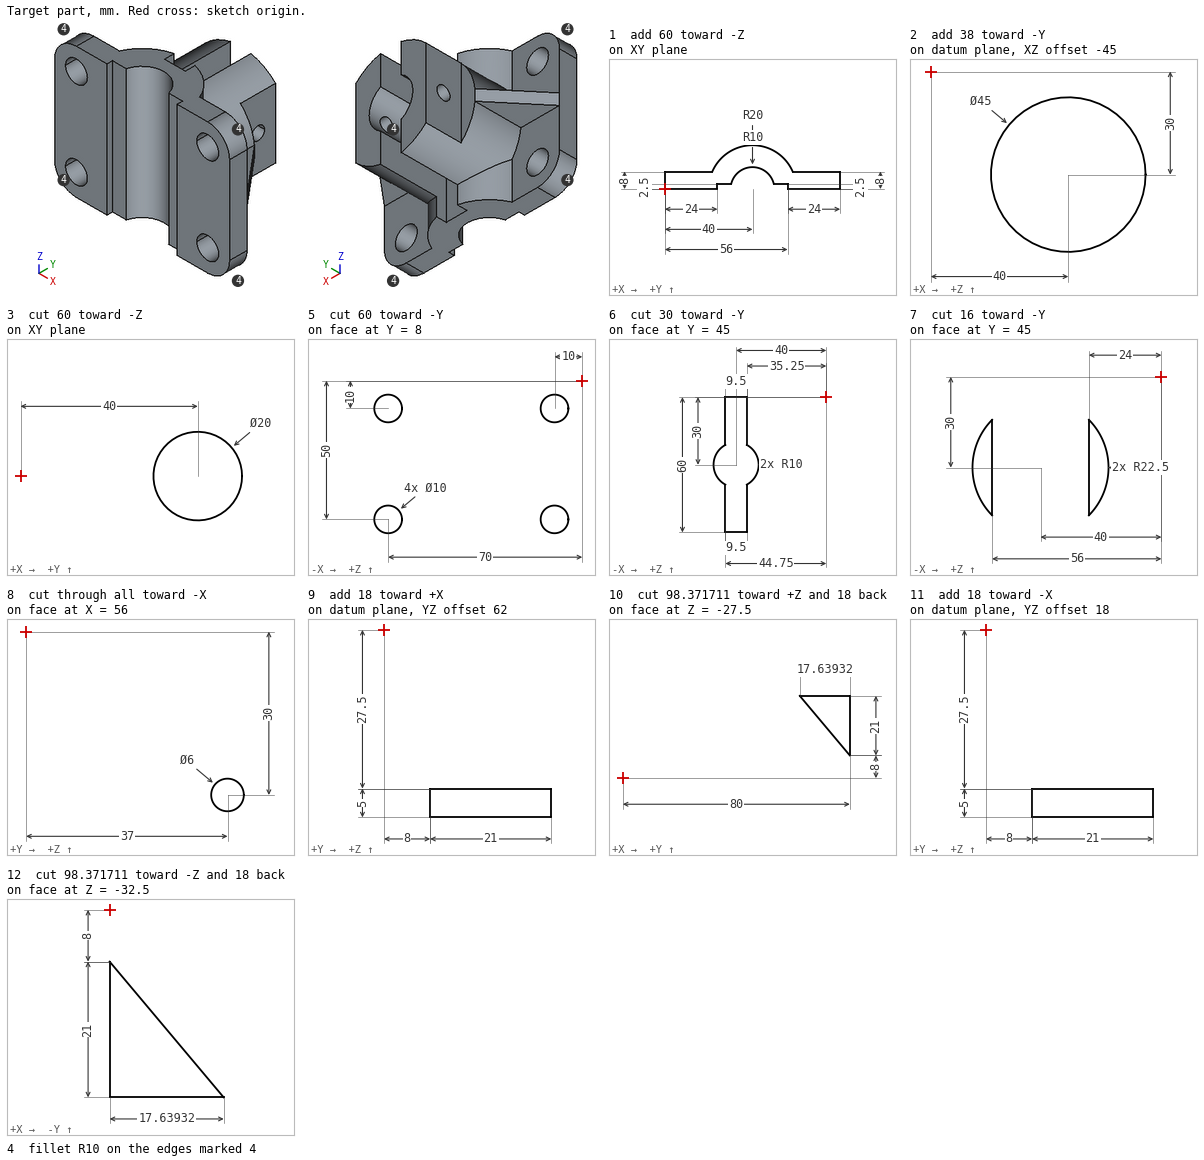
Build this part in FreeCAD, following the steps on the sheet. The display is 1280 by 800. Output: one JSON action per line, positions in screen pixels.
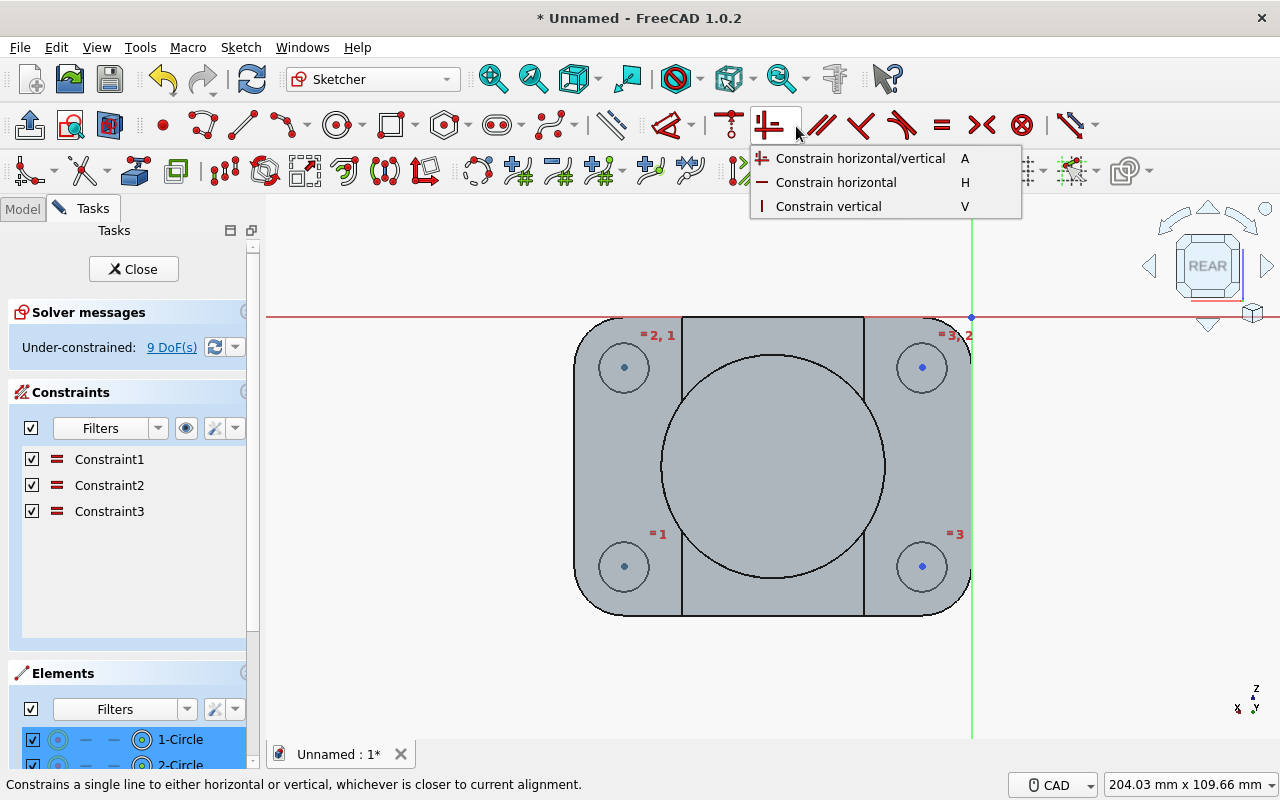
{"action": "left_click", "coordinate": [886, 206]}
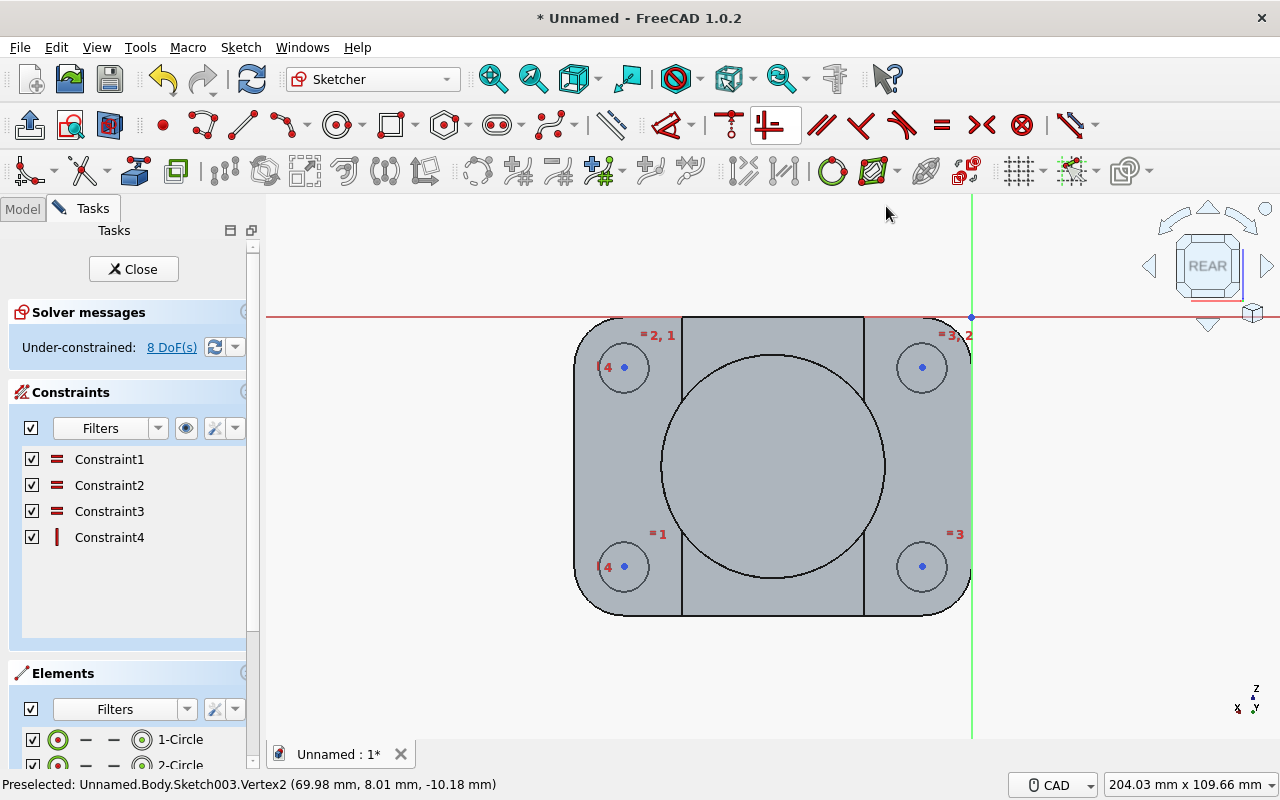
{"action": "left_click", "coordinate": [624, 368]}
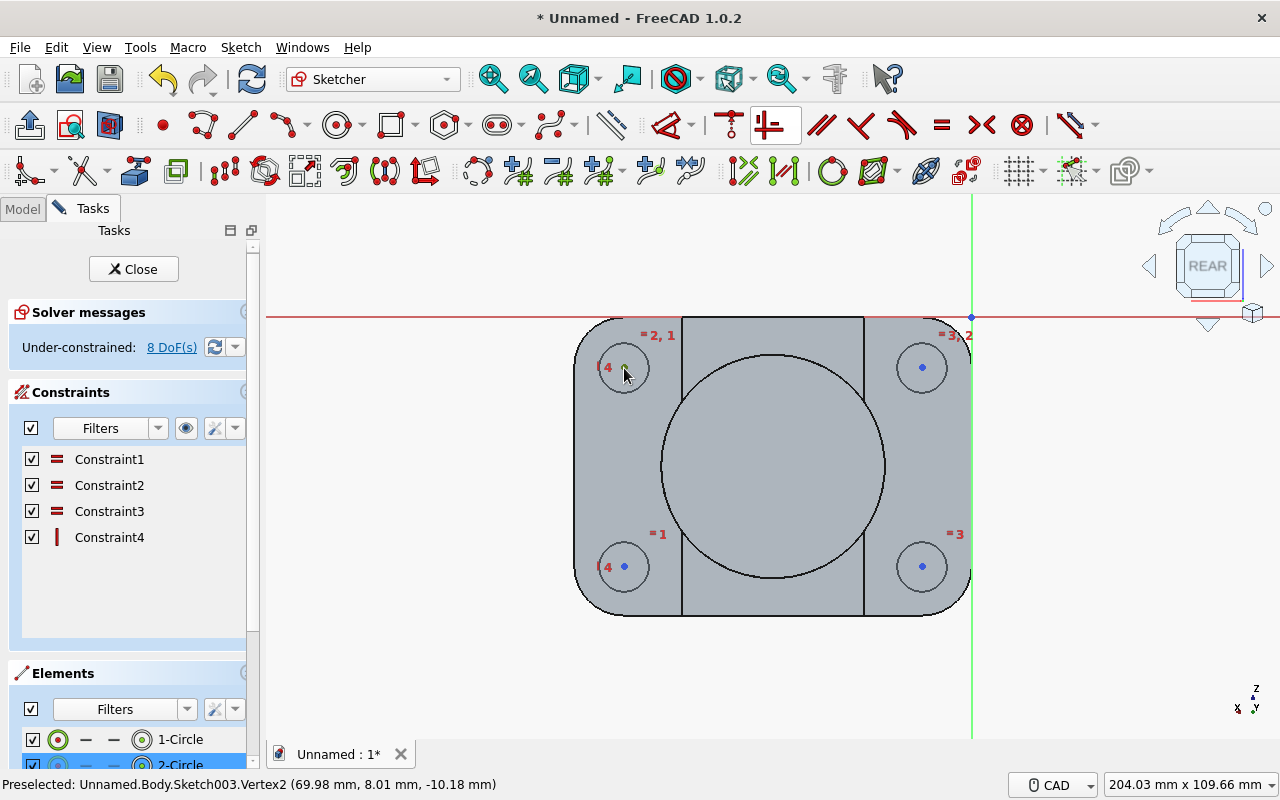
{"action": "left_click", "coordinate": [922, 368]}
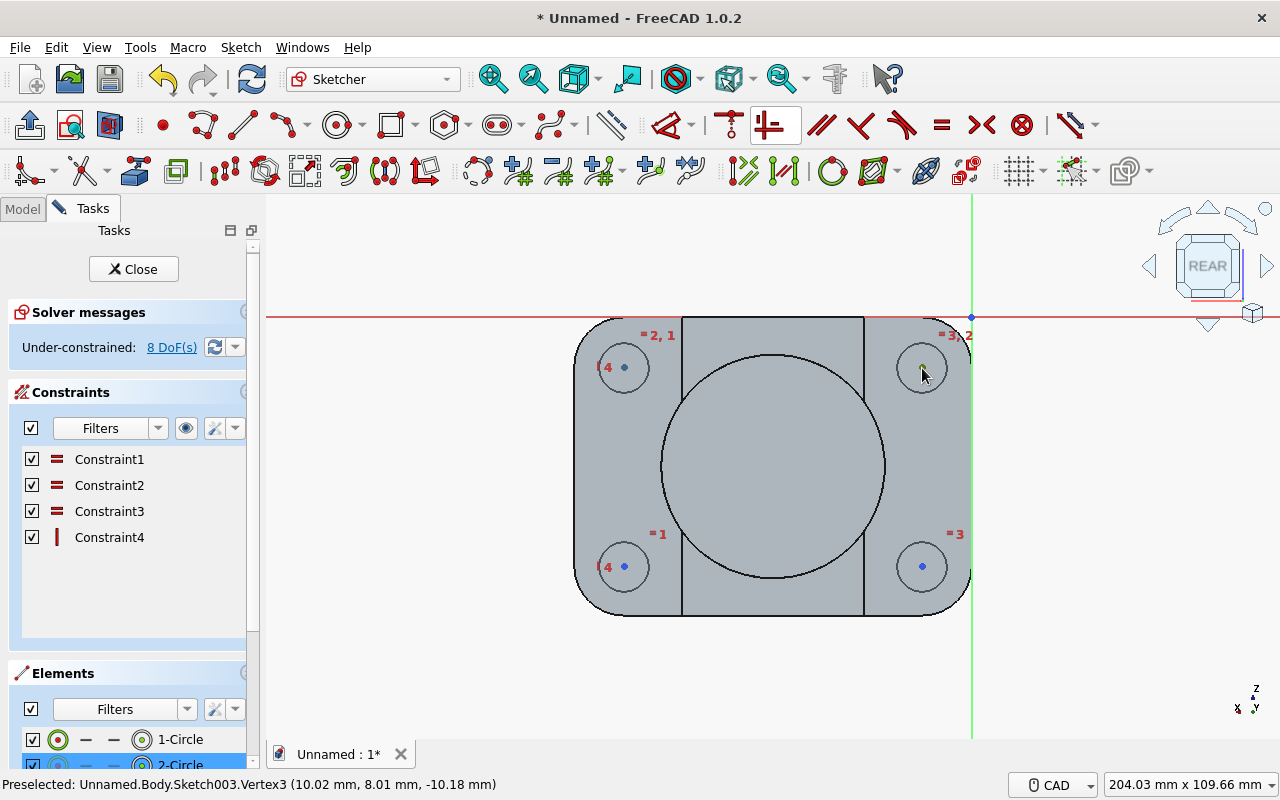
{"action": "left_click", "coordinate": [796, 126]}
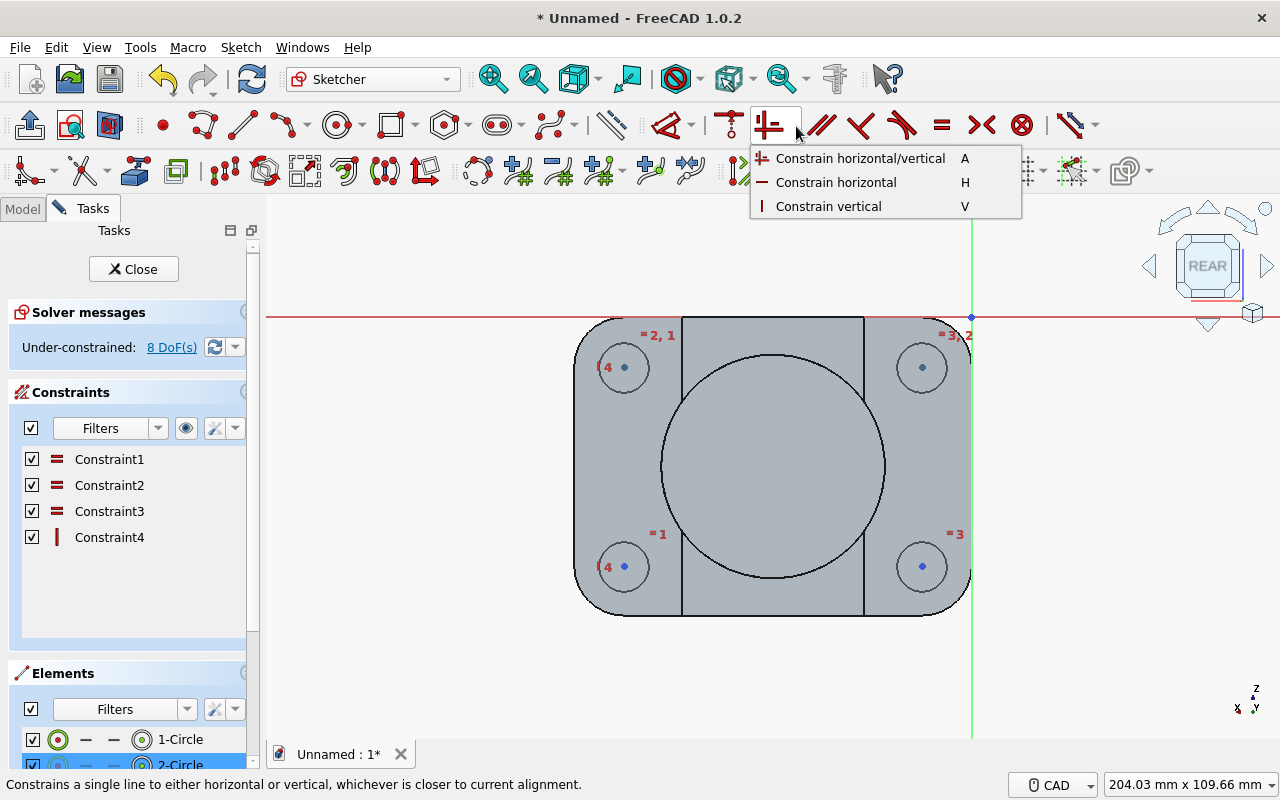
{"action": "left_click", "coordinate": [886, 182]}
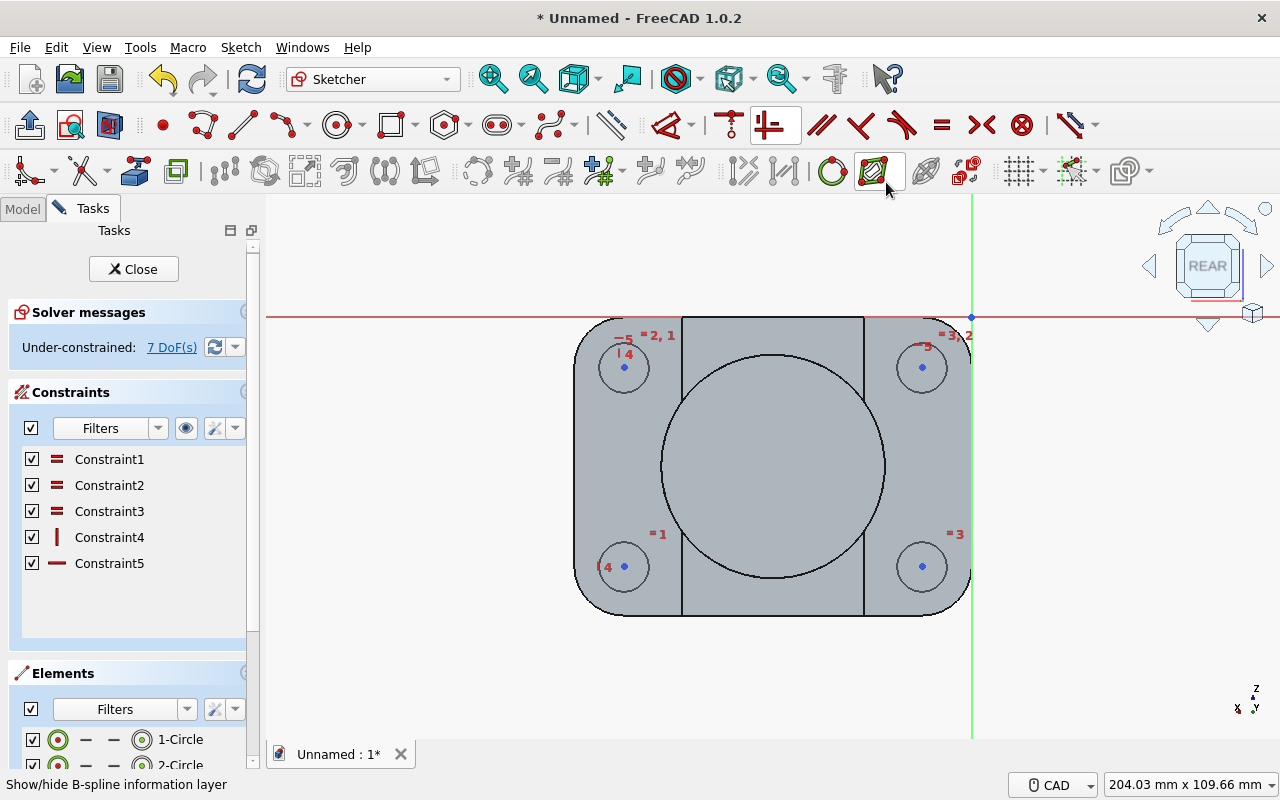
{"action": "left_click", "coordinate": [922, 368]}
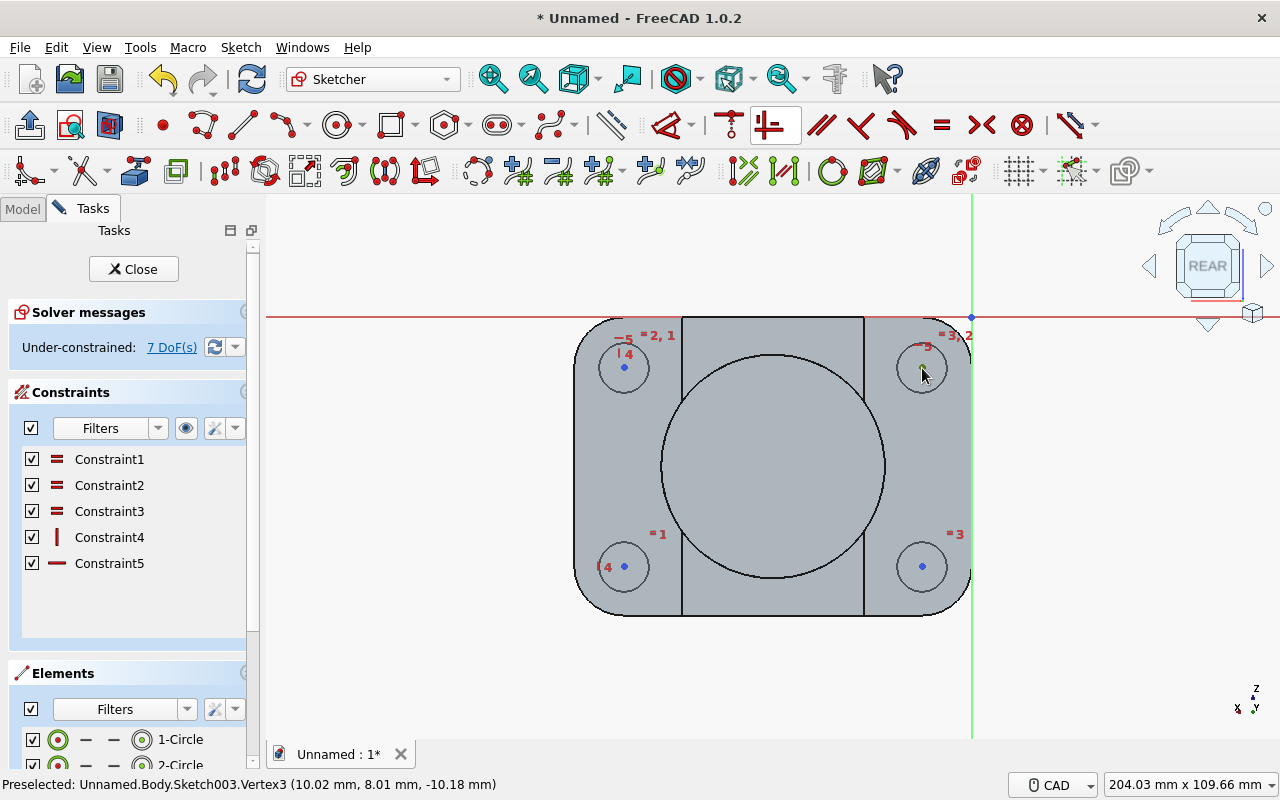
{"action": "left_click", "coordinate": [922, 567]}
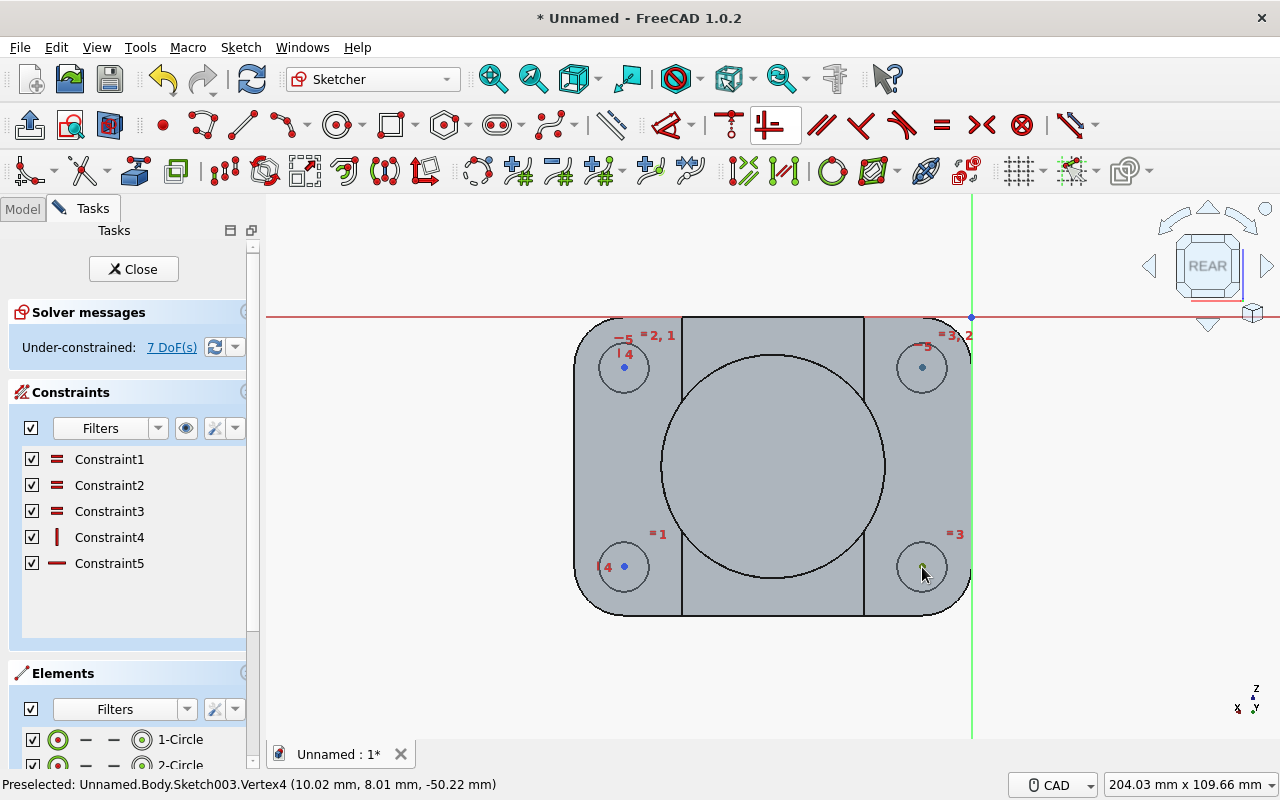
{"action": "left_click", "coordinate": [796, 126]}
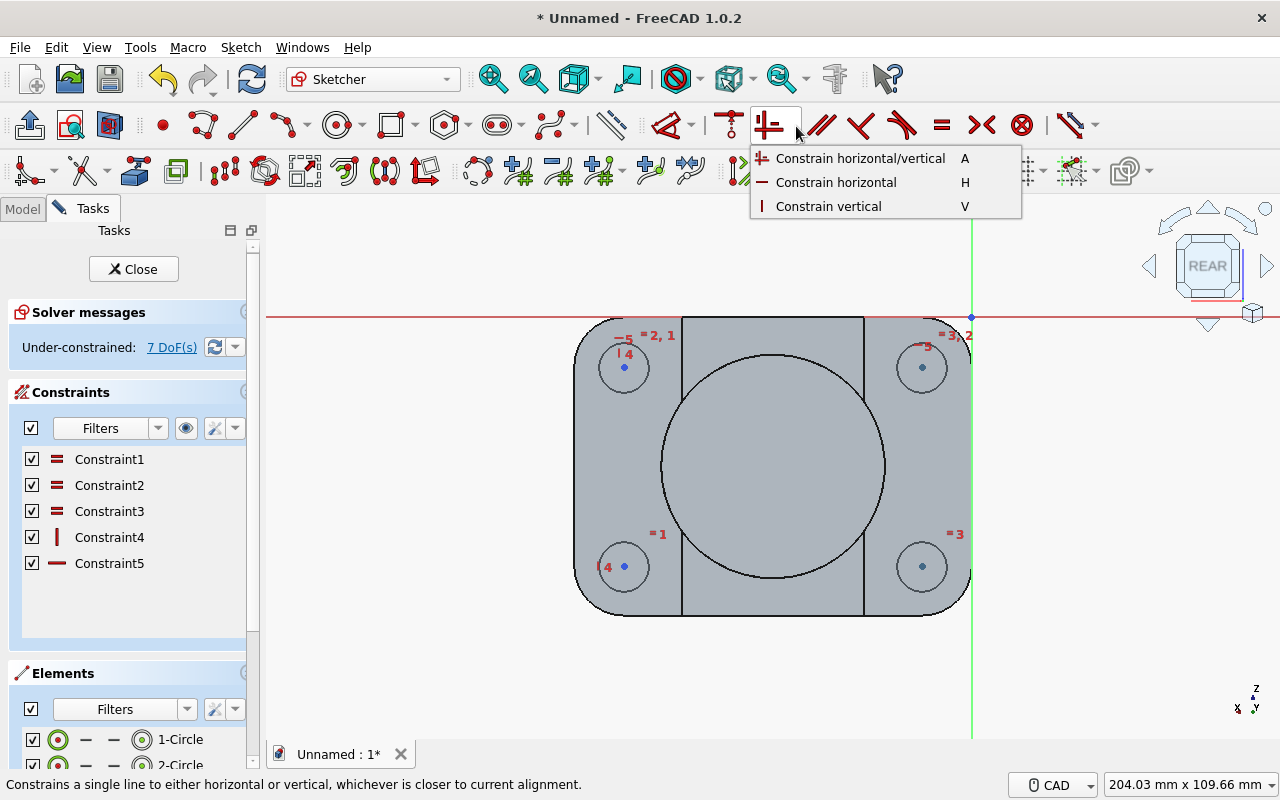
{"action": "left_click", "coordinate": [886, 206]}